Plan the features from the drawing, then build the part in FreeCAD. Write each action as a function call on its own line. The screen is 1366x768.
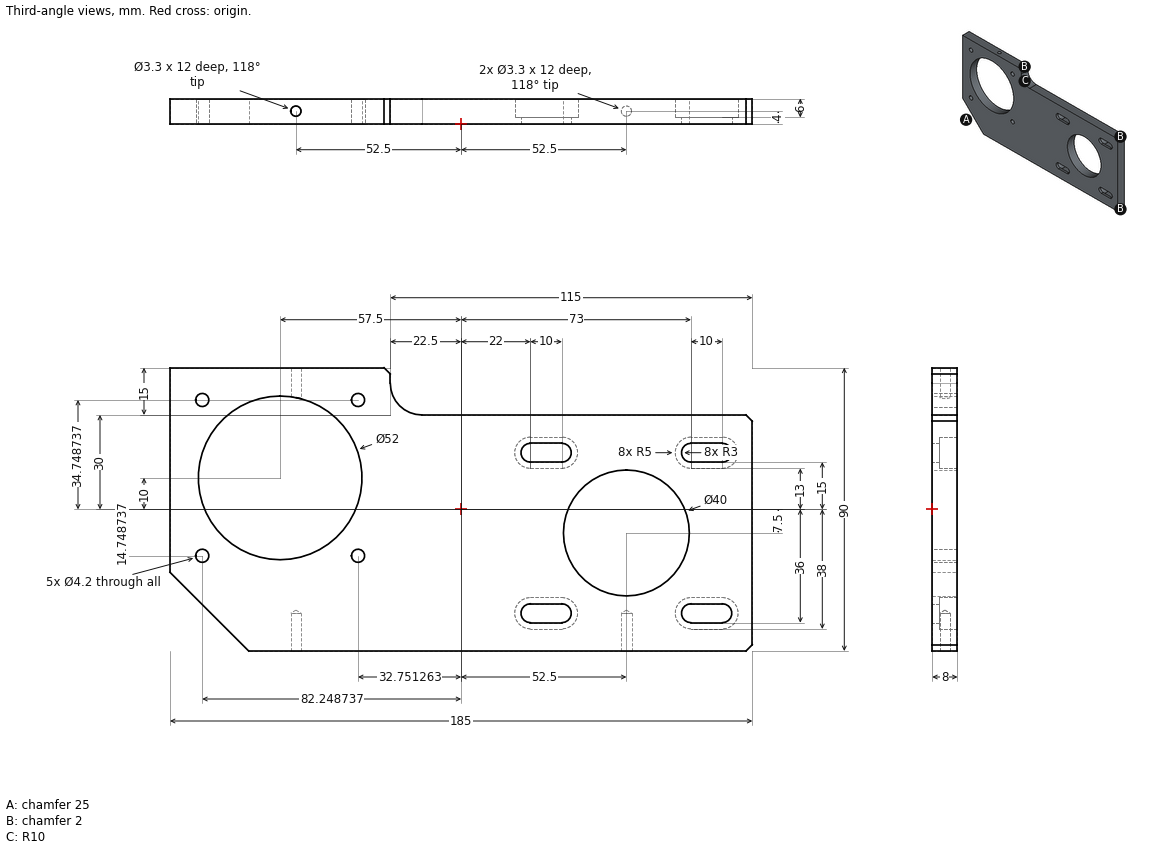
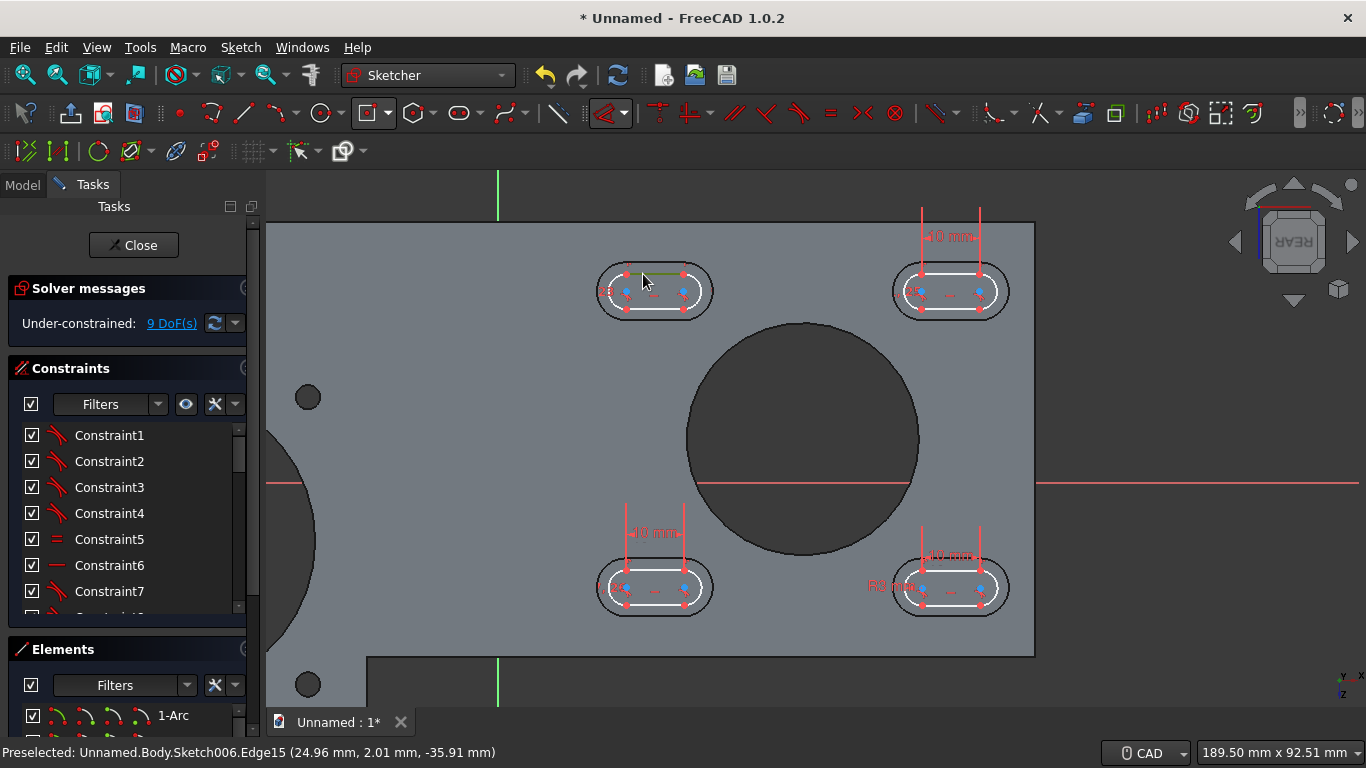
key(l)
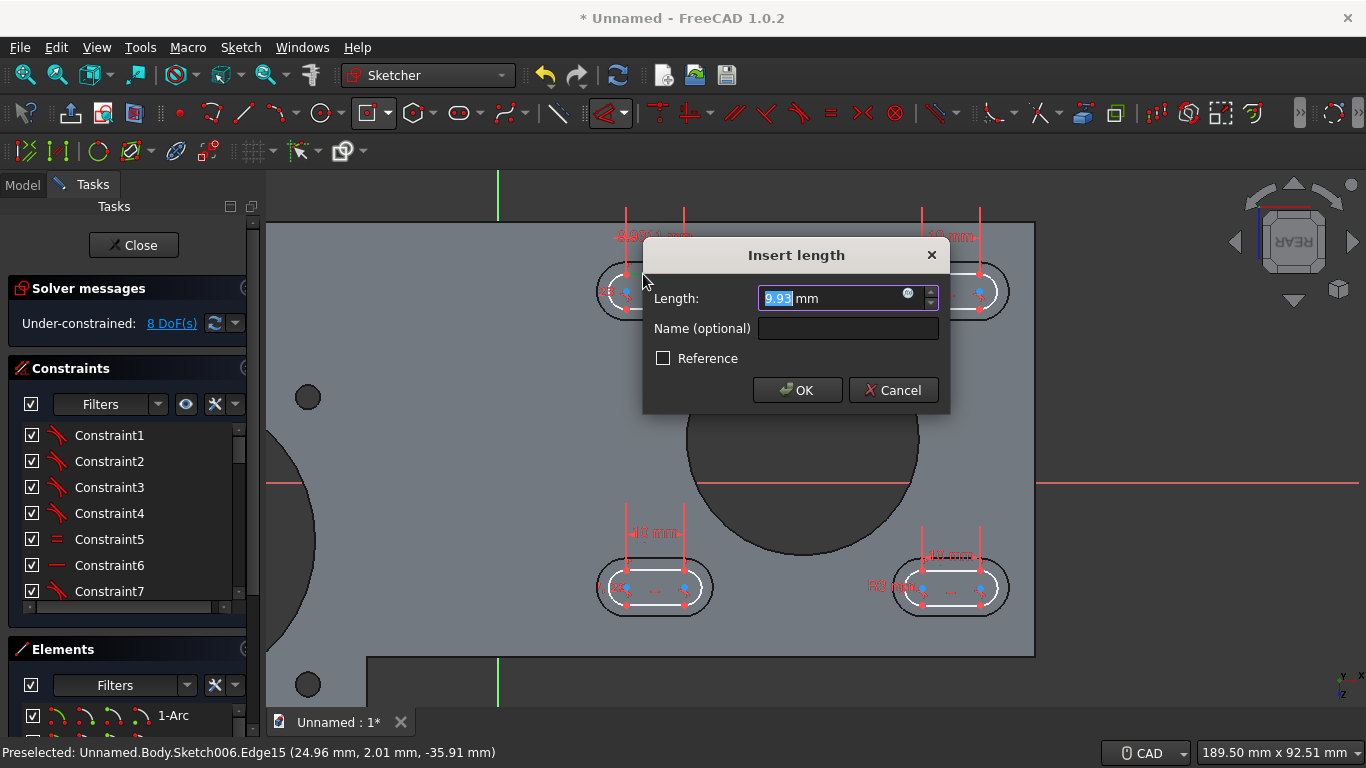
text(10)
key(Return)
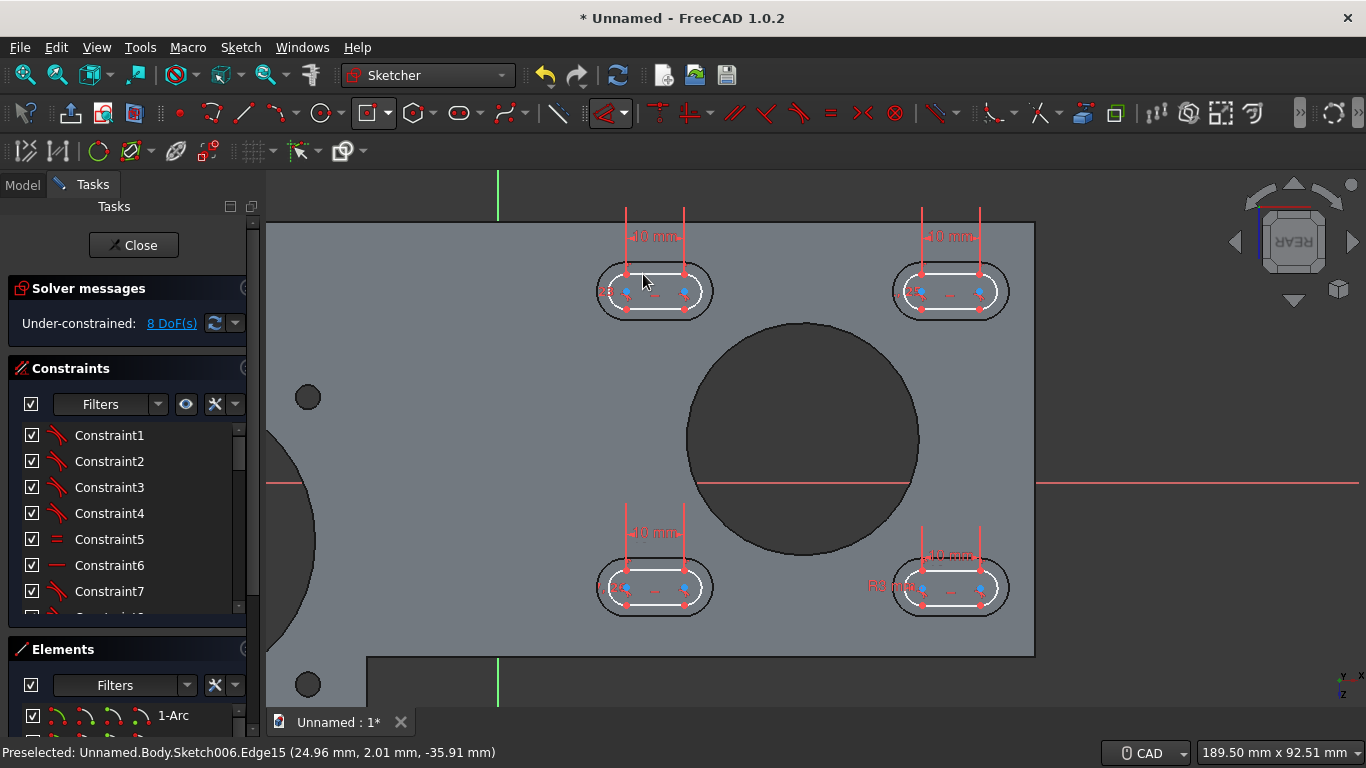
click(922, 571)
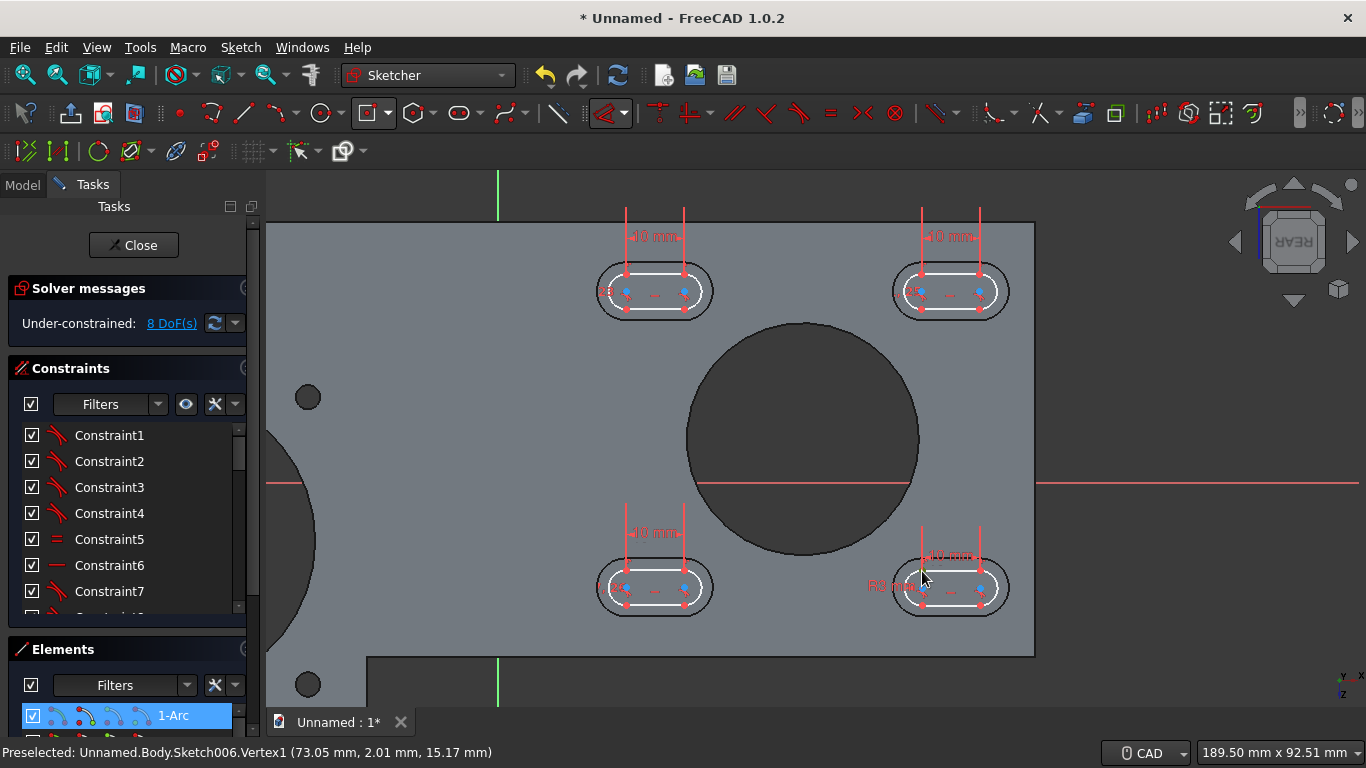
key(l)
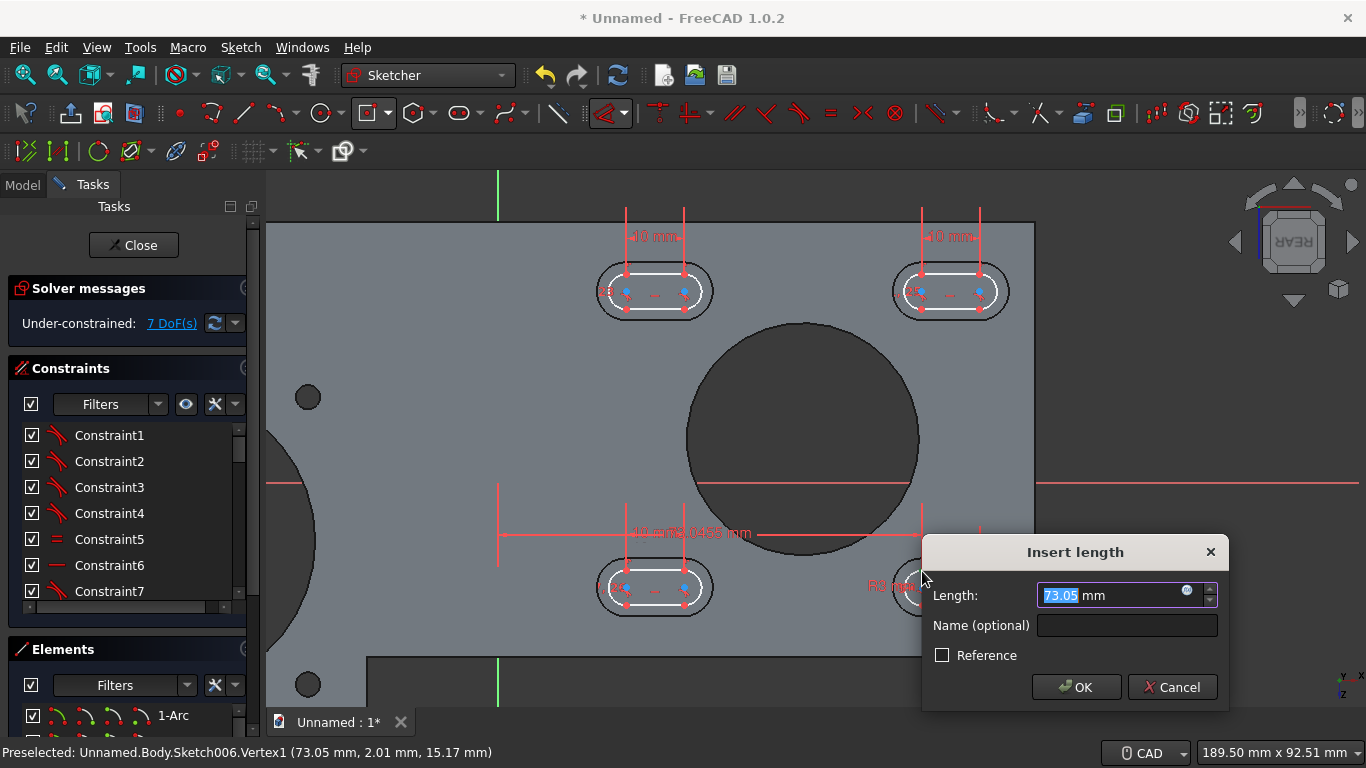
text(73)
key(Return)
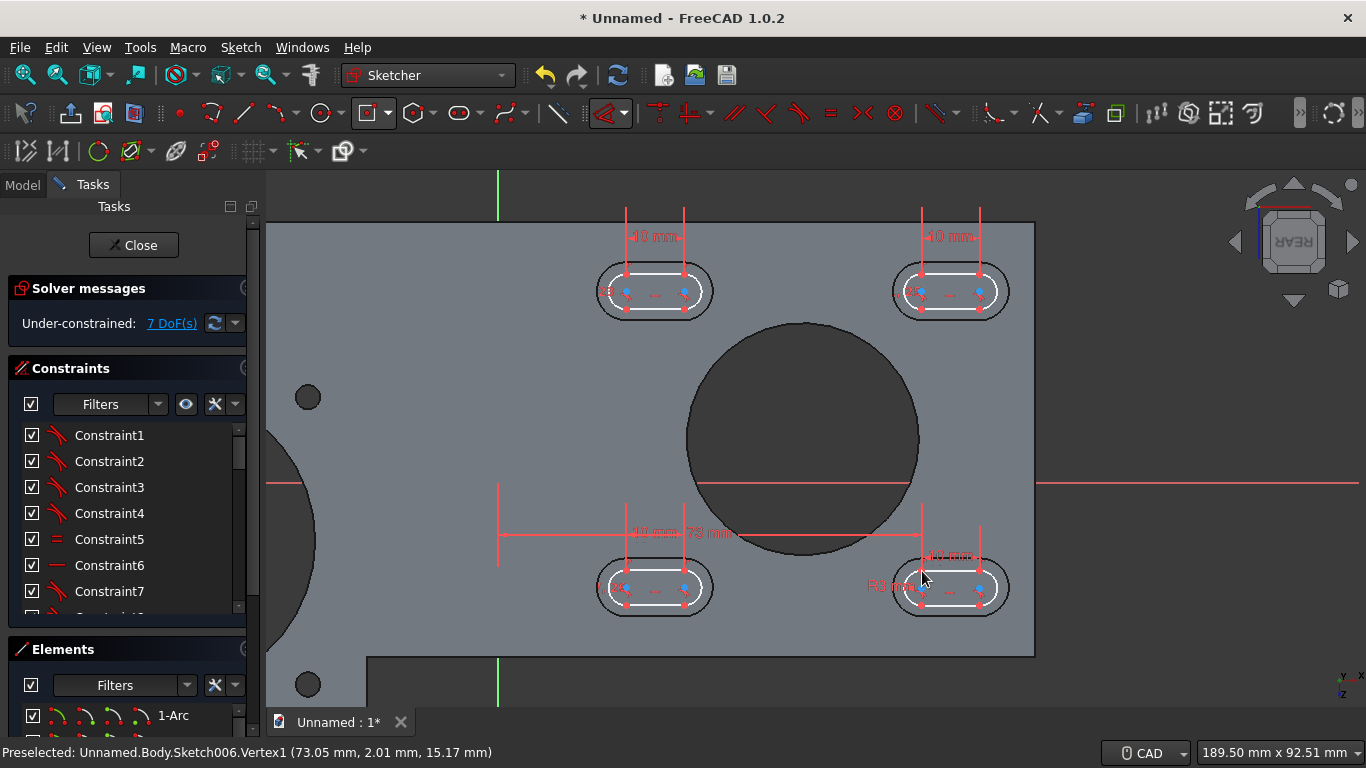
click(922, 571)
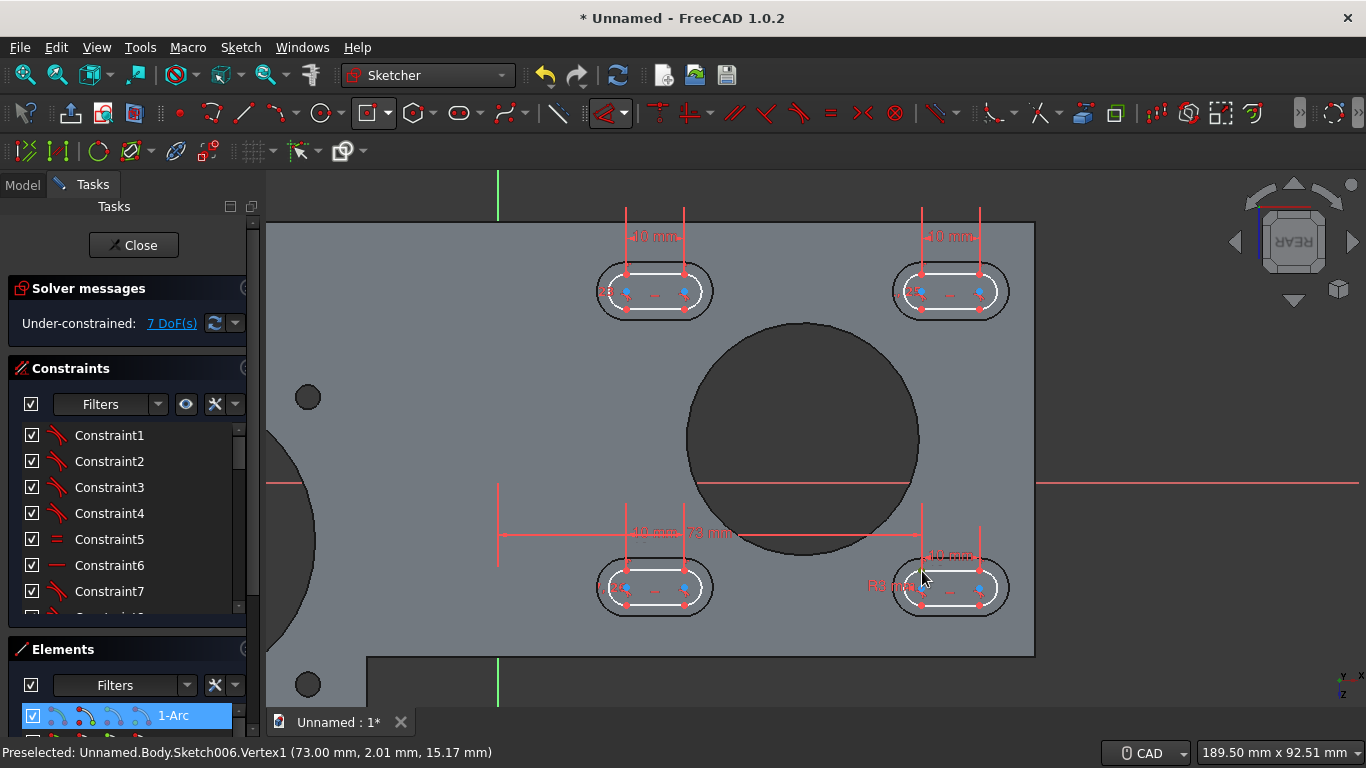
key(i)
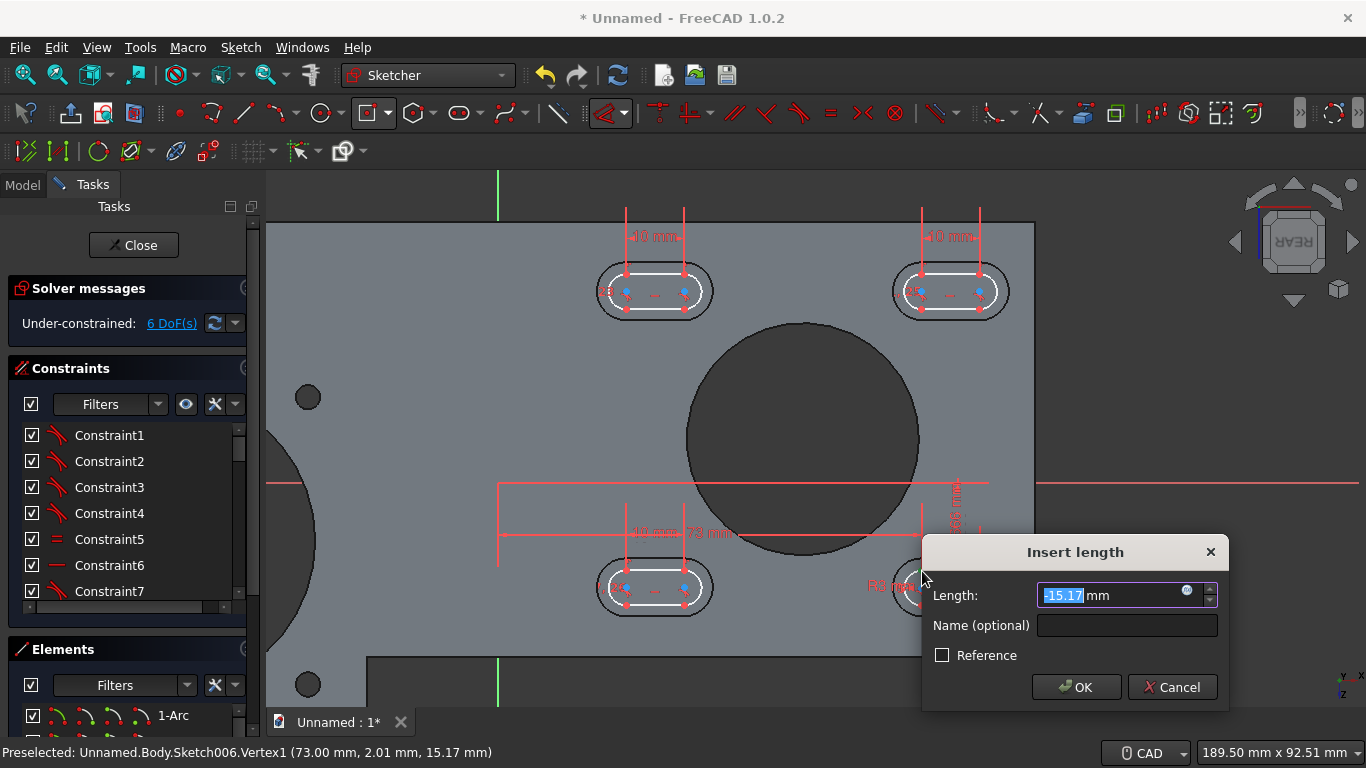
text(-15)
key(Return)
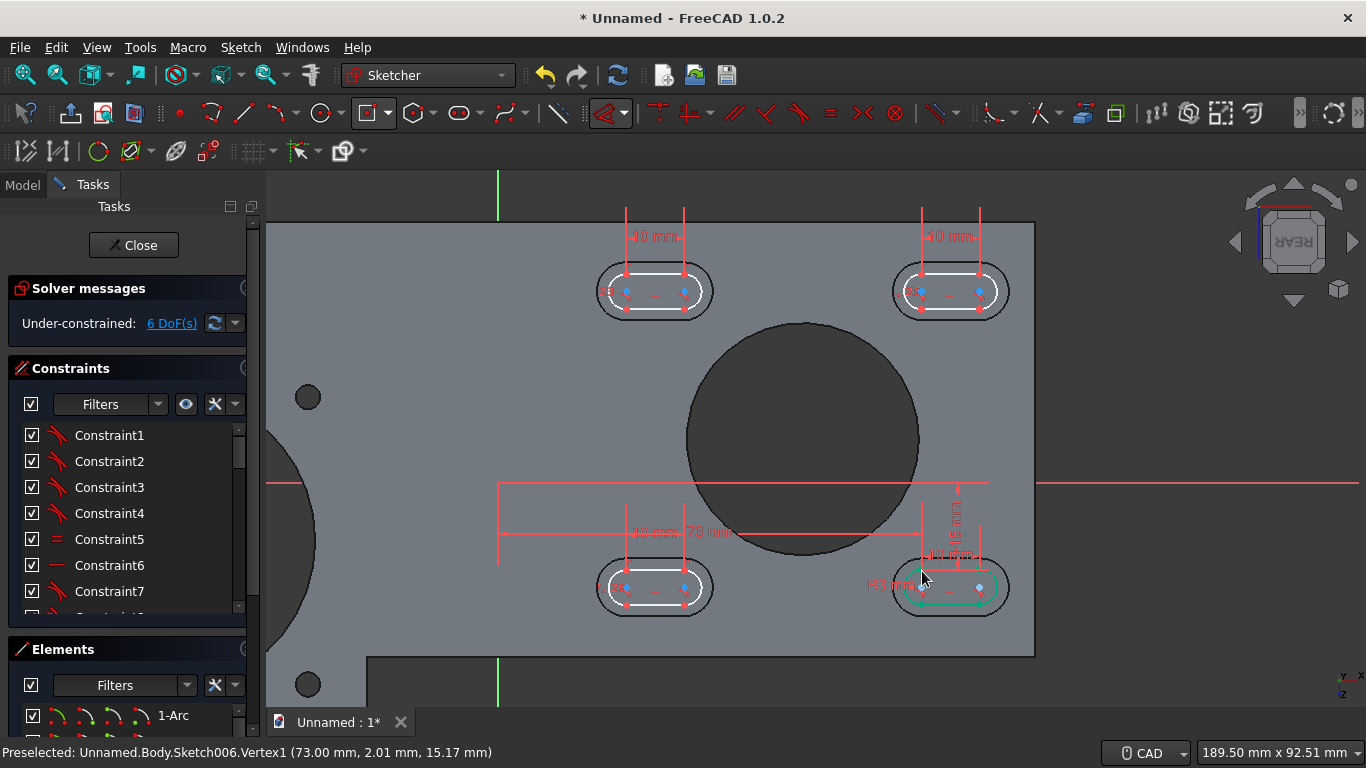
click(922, 274)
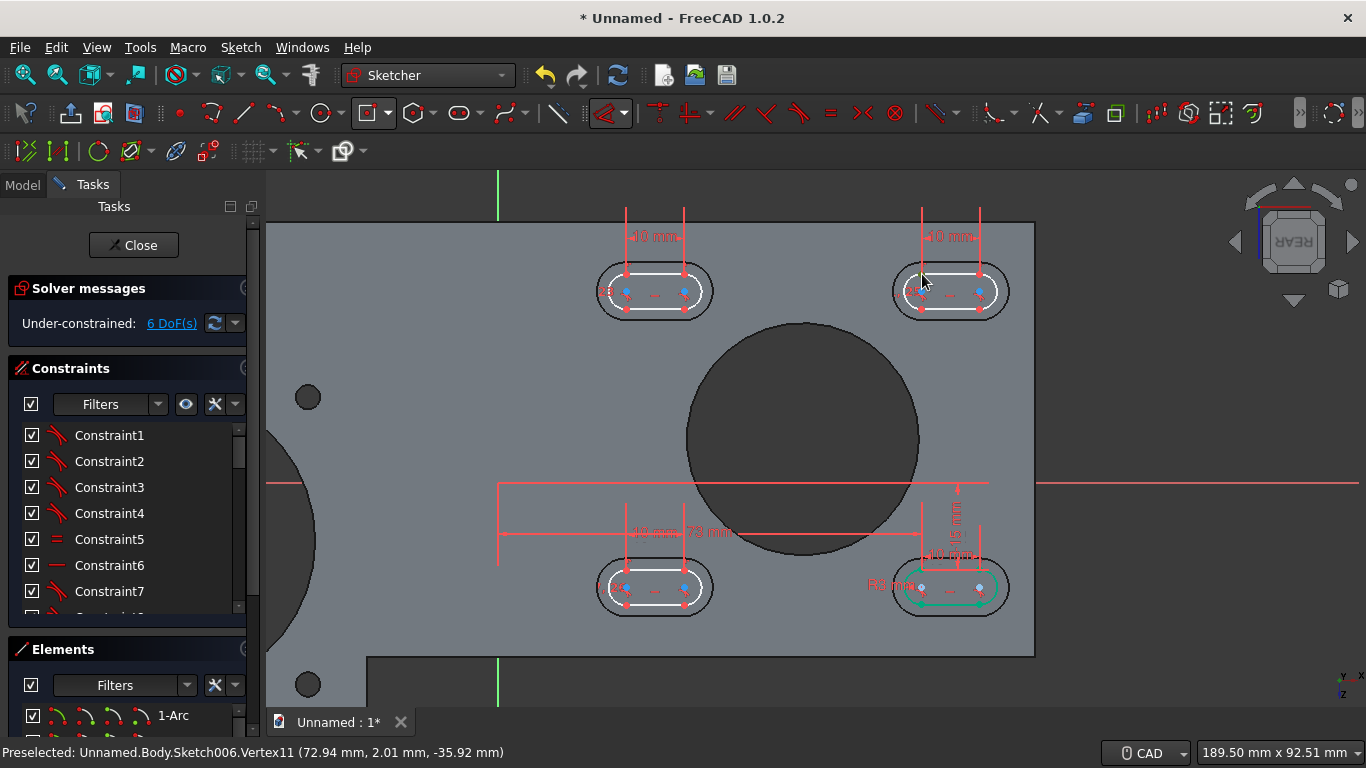
click(626, 114)